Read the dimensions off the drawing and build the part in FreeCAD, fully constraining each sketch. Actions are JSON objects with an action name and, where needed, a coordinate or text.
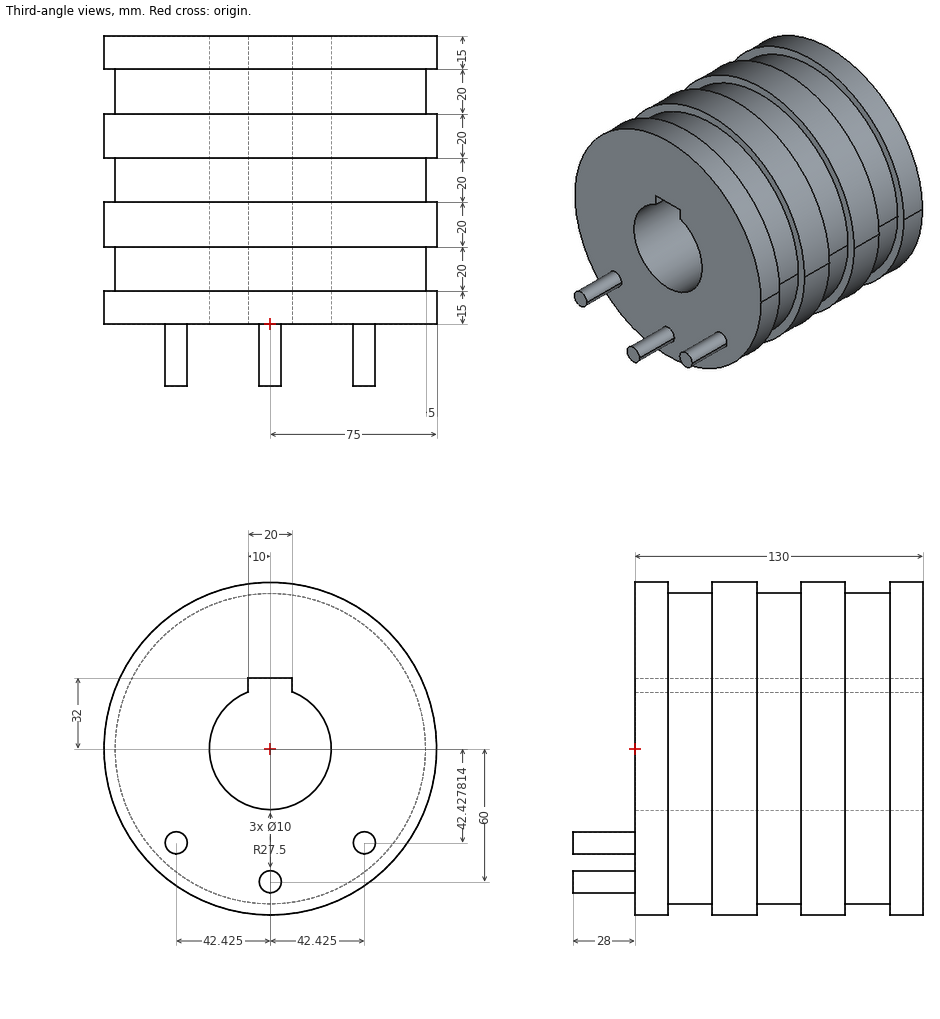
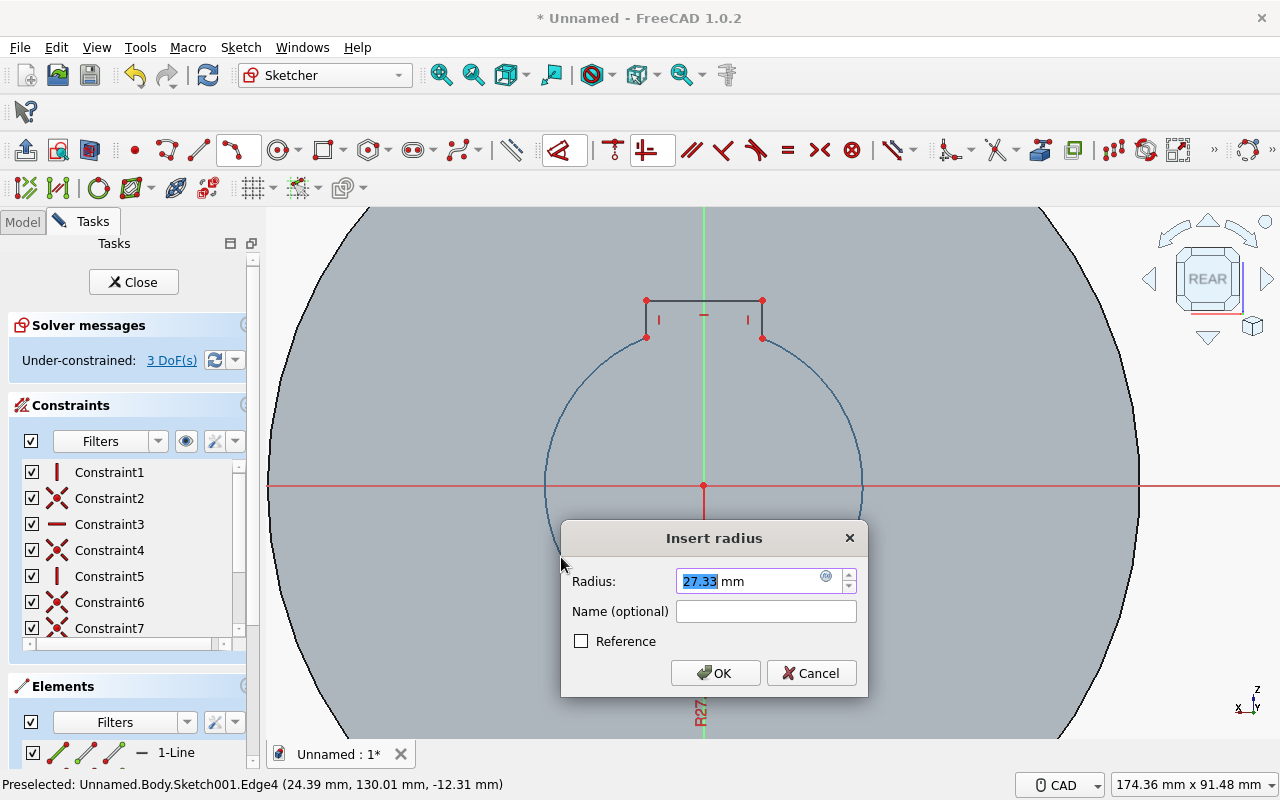
{"action": "type", "text": "27.5"}
{"action": "key", "text": "Return"}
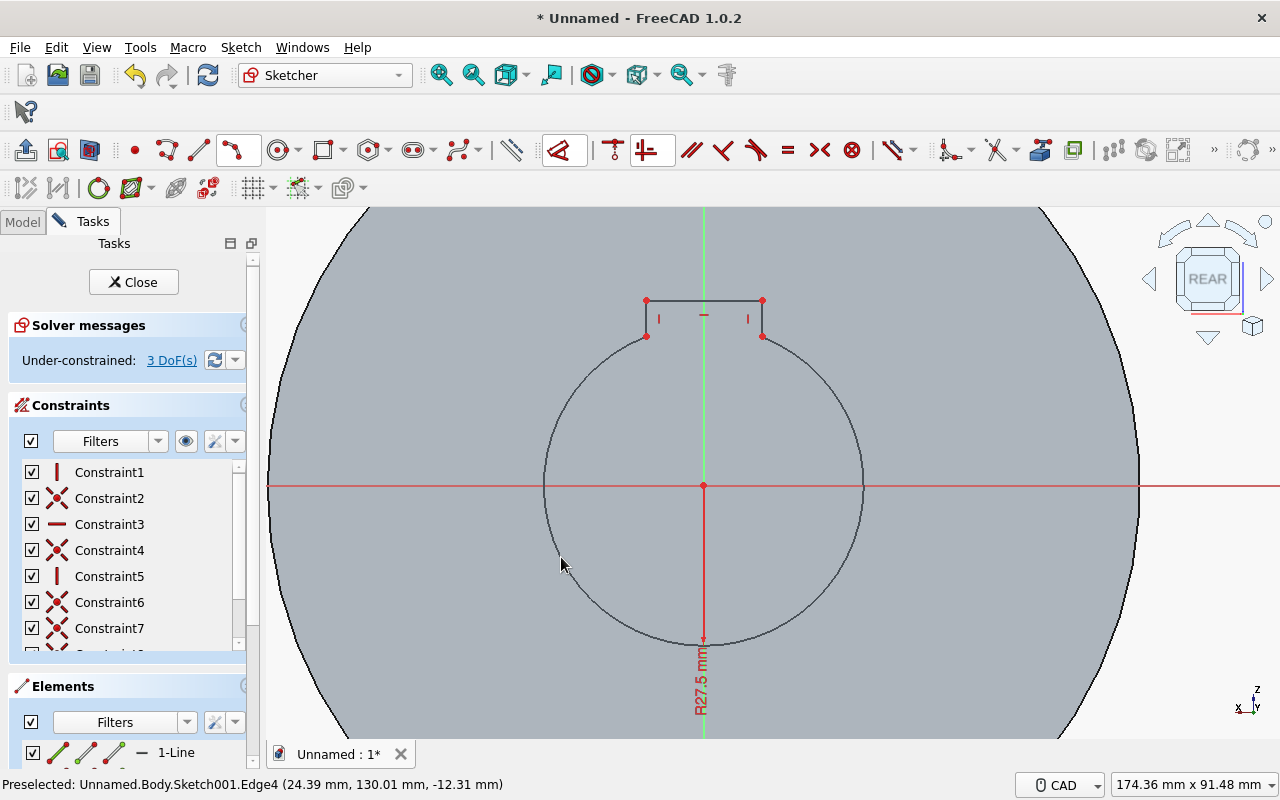
{"action": "left_click", "coordinate": [727, 301]}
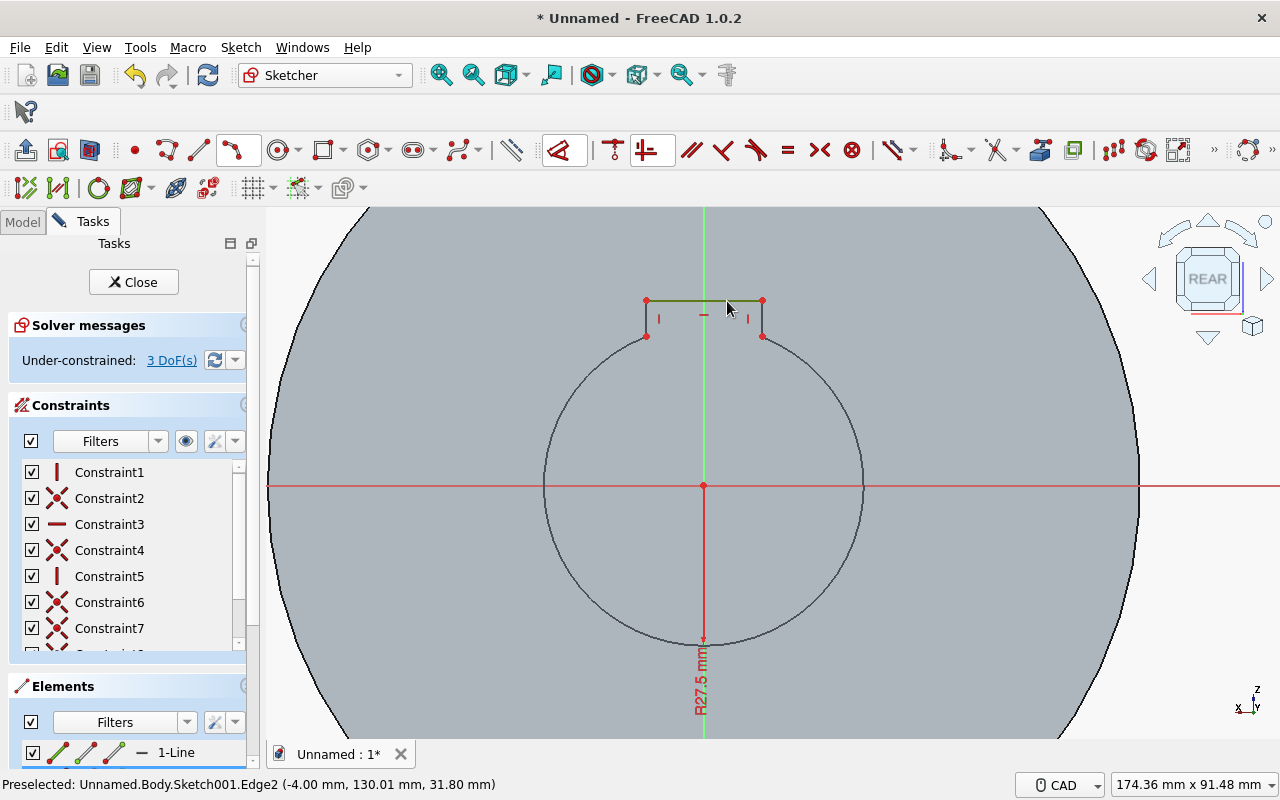
{"action": "key", "text": "l"}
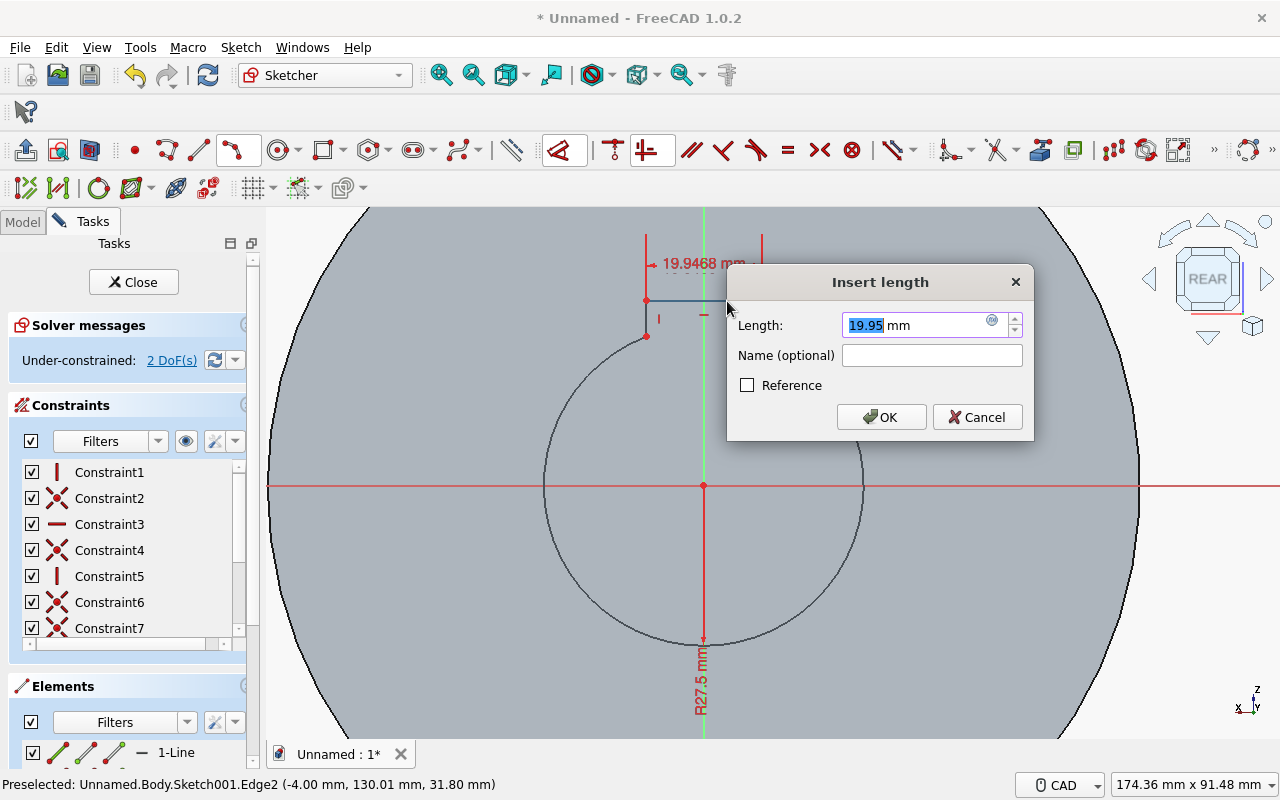
{"action": "type", "text": "20"}
{"action": "key", "text": "Return"}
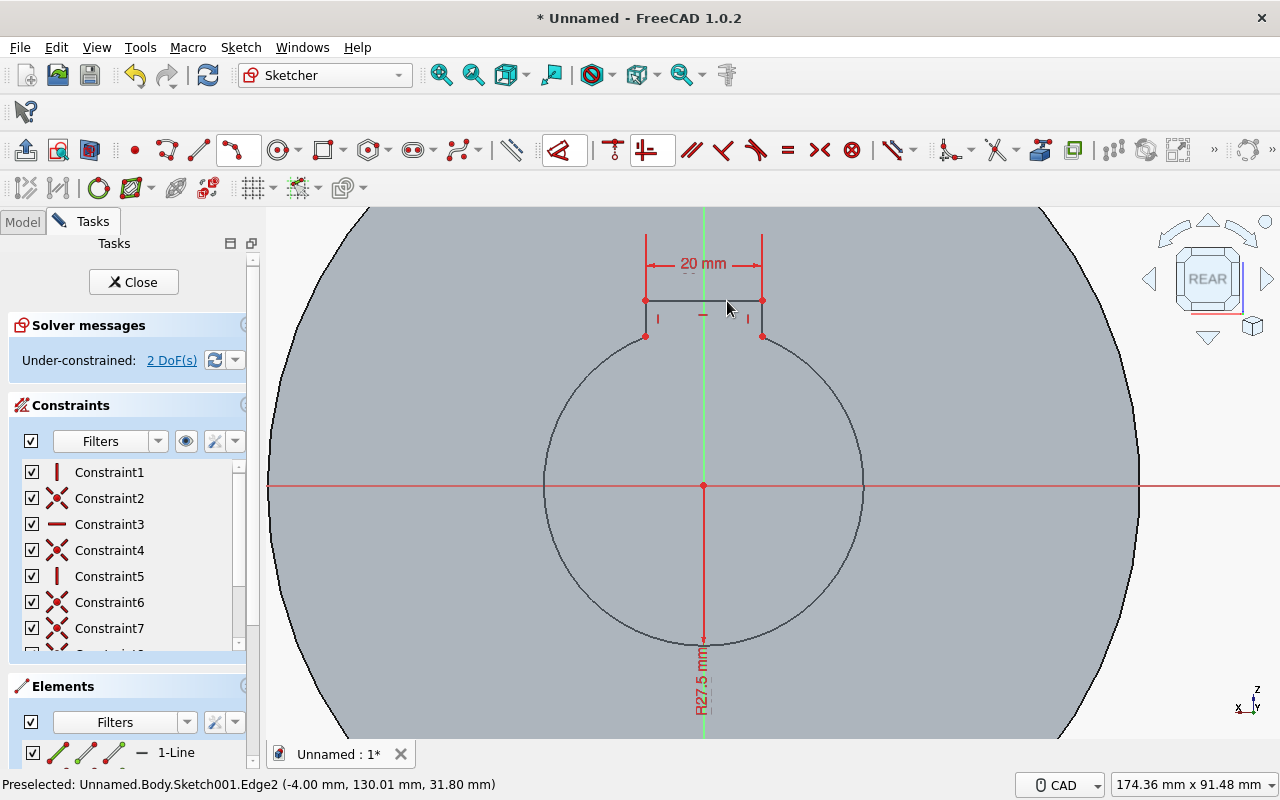
{"action": "left_click", "coordinate": [762, 337]}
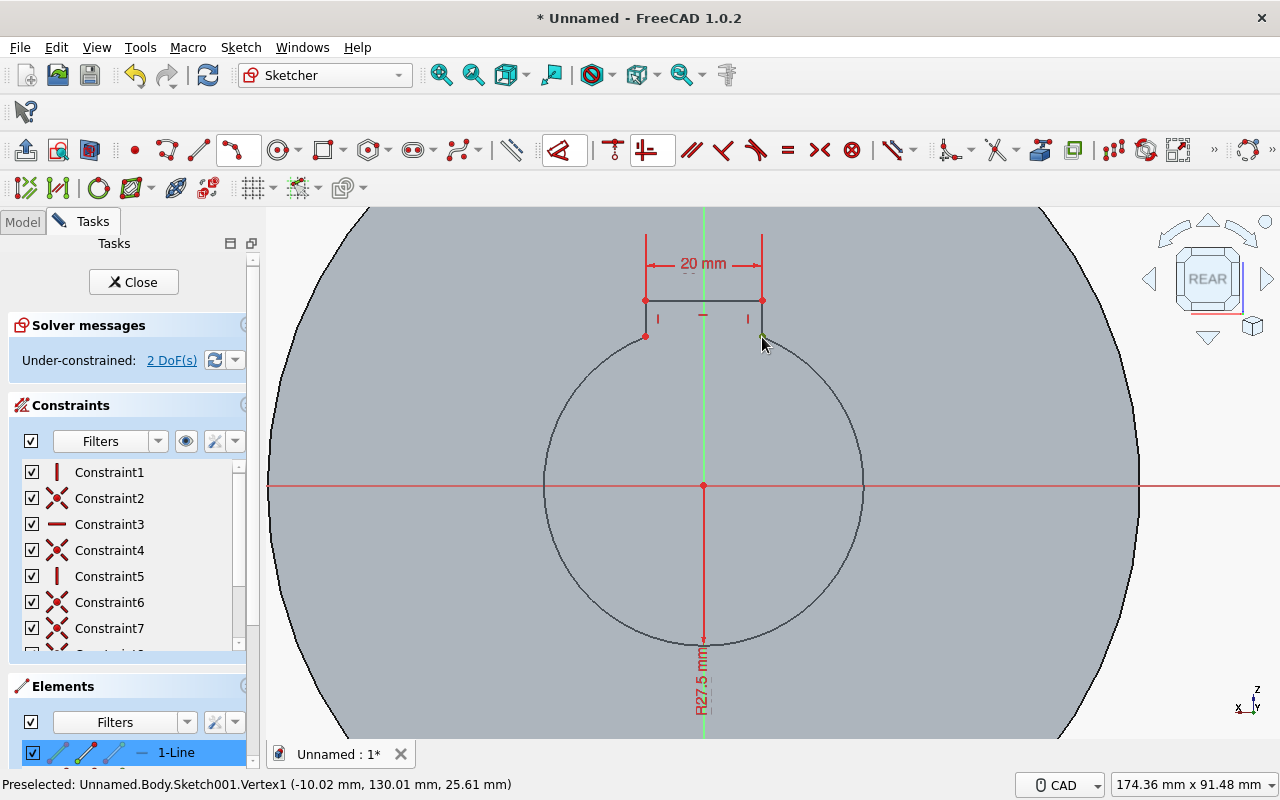
{"action": "key", "text": "l"}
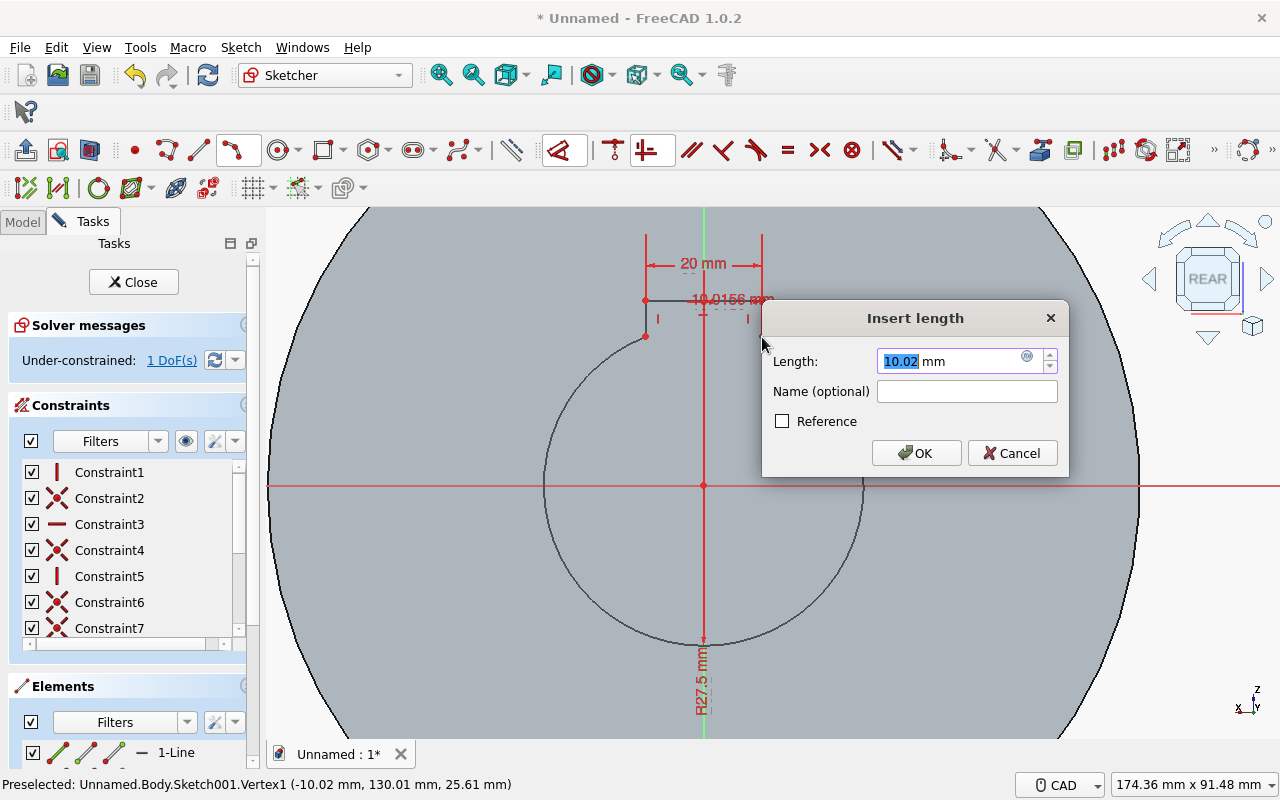
{"action": "type", "text": "10"}
{"action": "key", "text": "Return"}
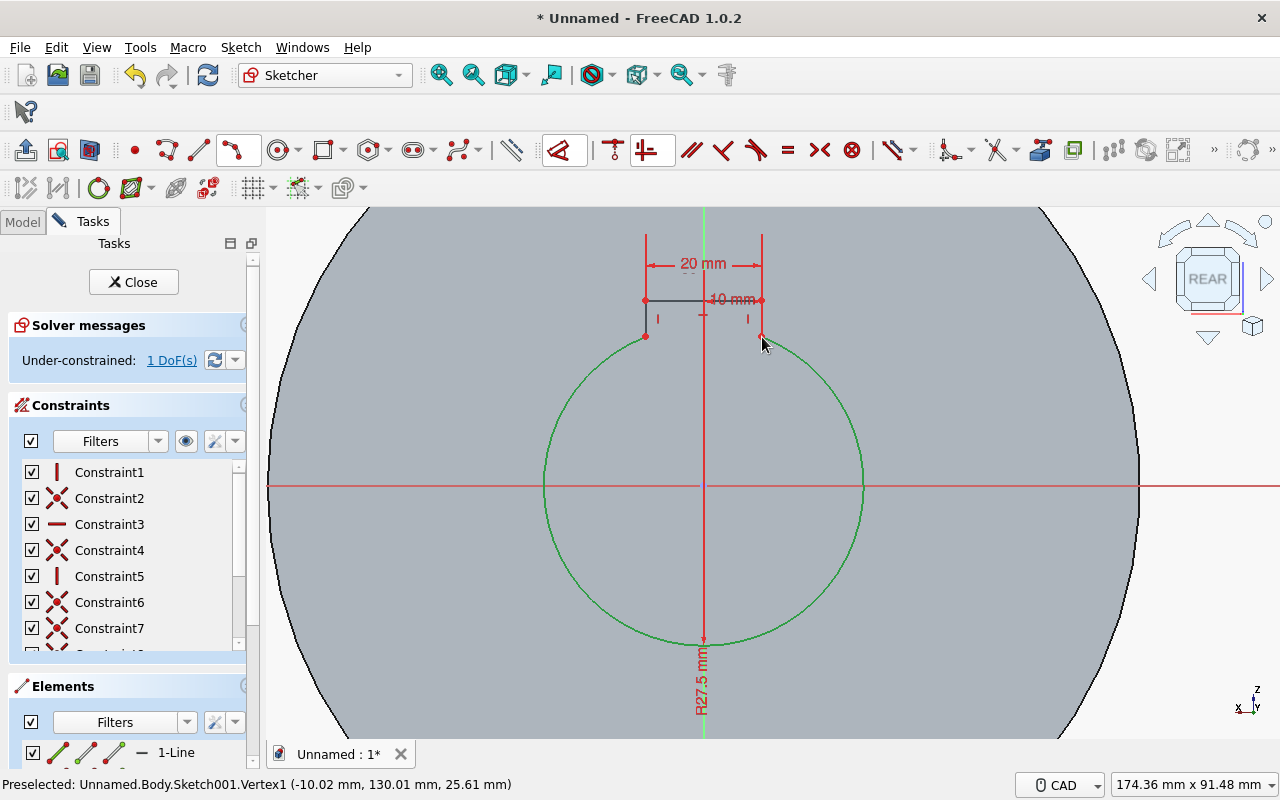
{"action": "left_click", "coordinate": [762, 301]}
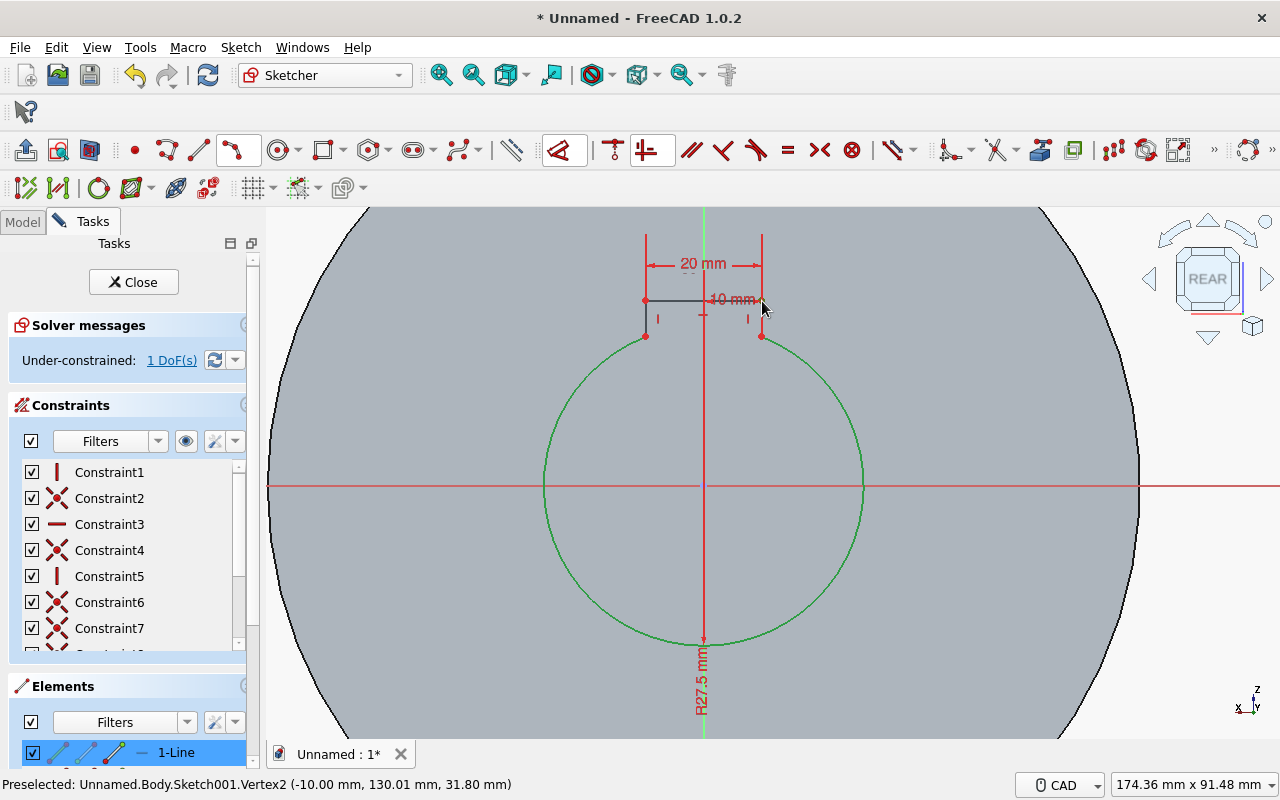
{"action": "key", "text": "i"}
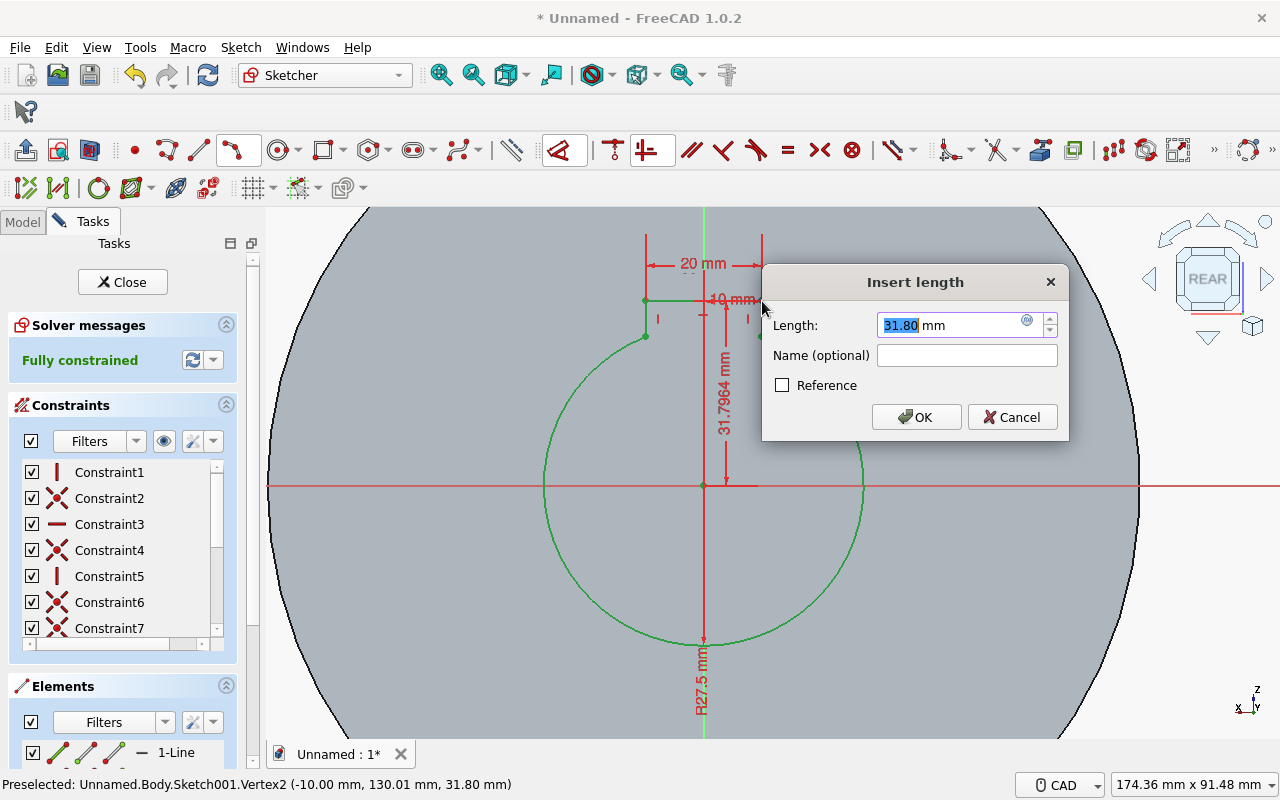
{"action": "type", "text": "32"}
{"action": "key", "text": "Return"}